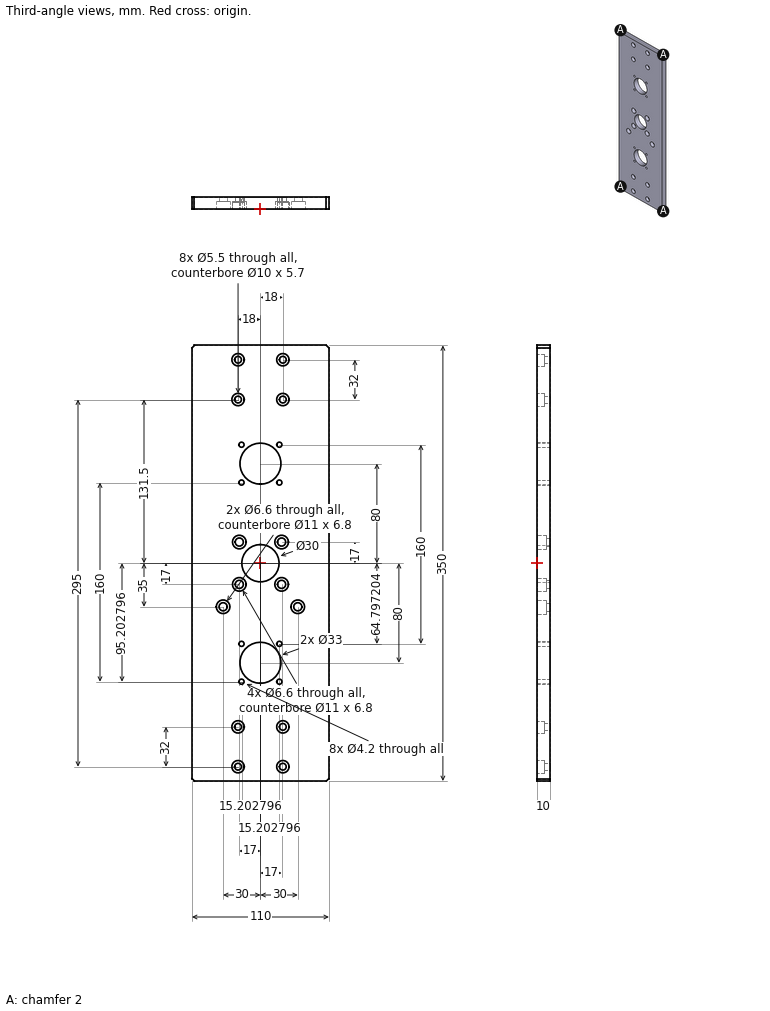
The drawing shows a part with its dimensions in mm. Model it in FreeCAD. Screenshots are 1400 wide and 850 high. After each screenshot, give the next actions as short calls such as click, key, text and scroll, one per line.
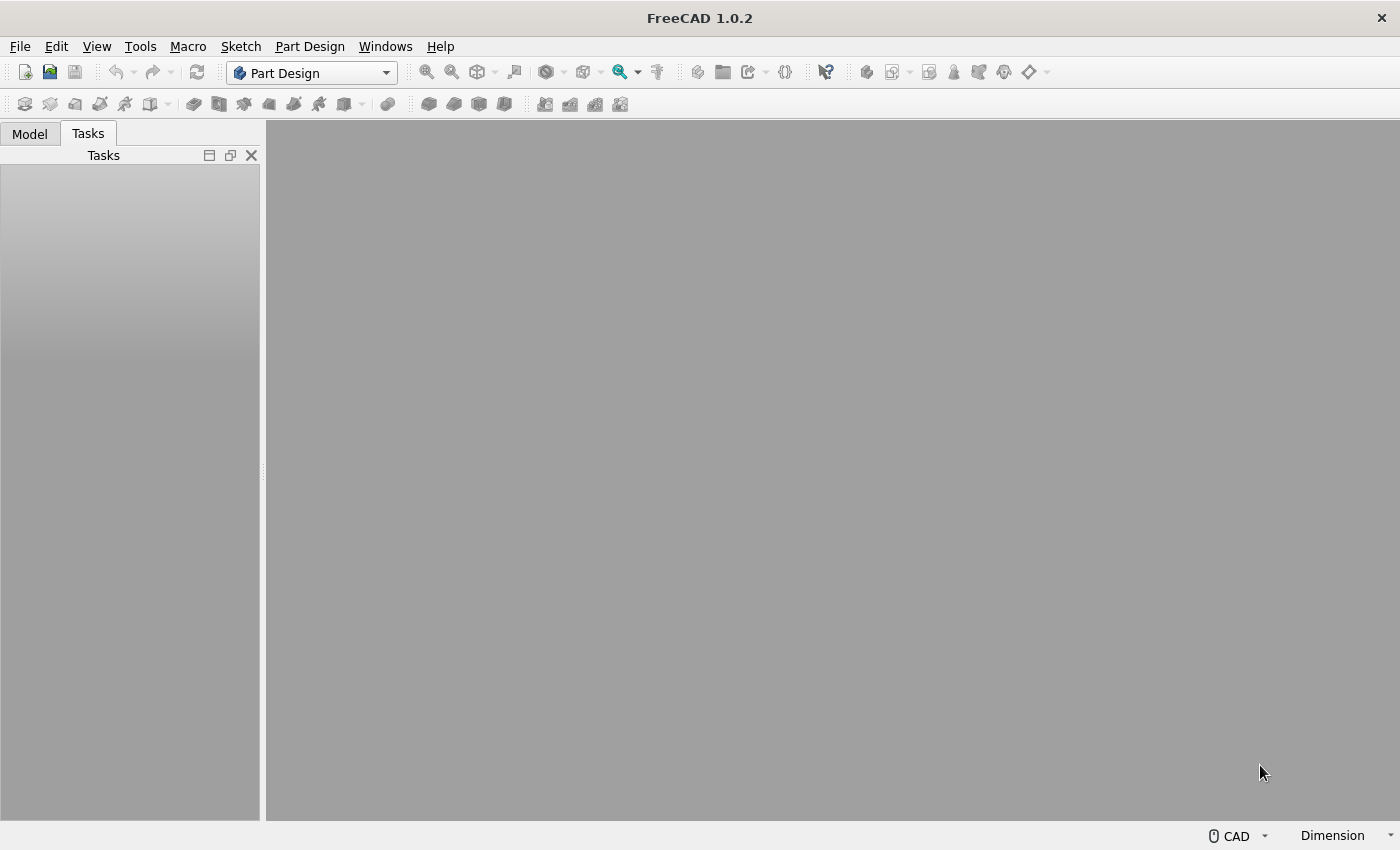
key(ctrl+n)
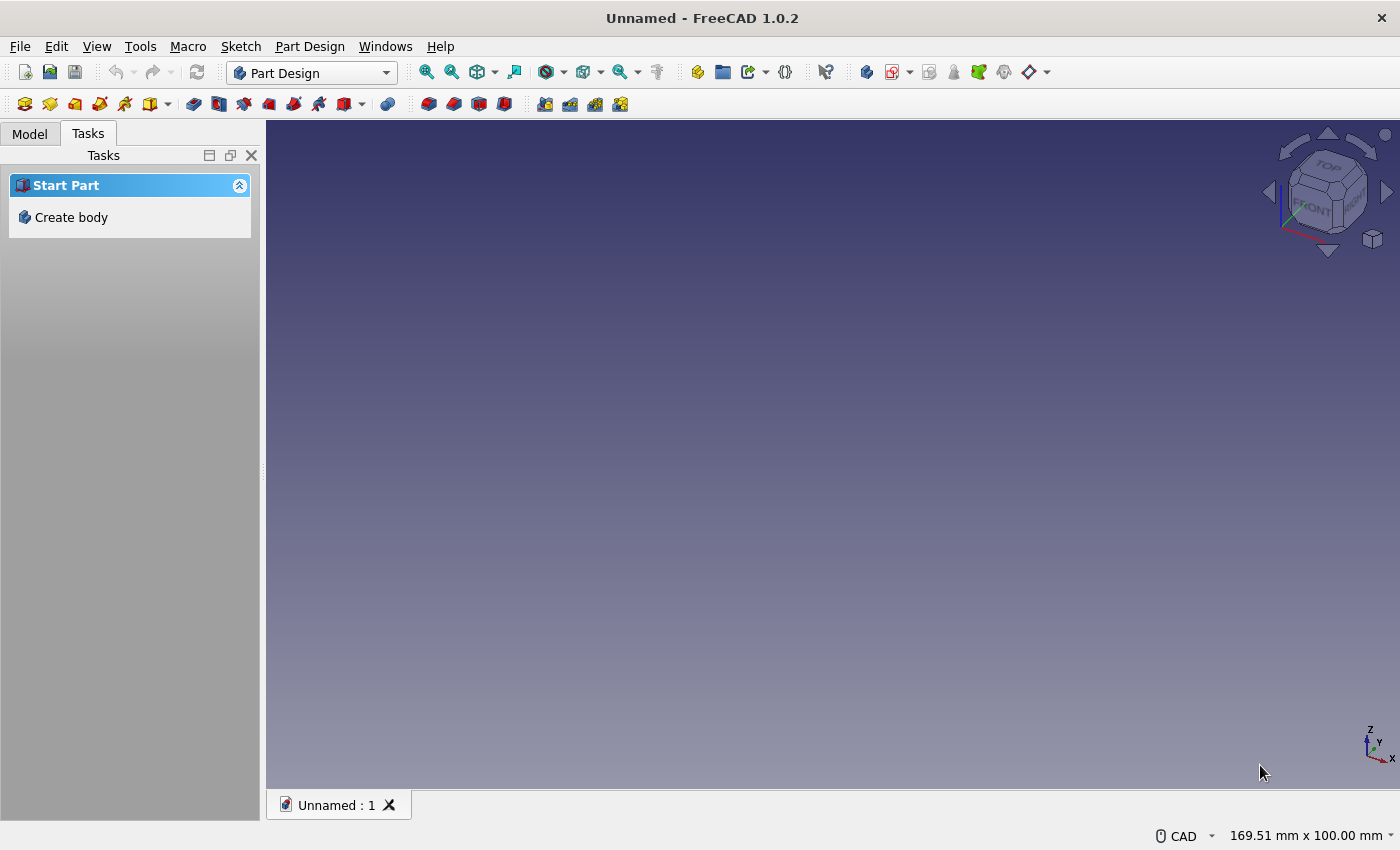
click(892, 72)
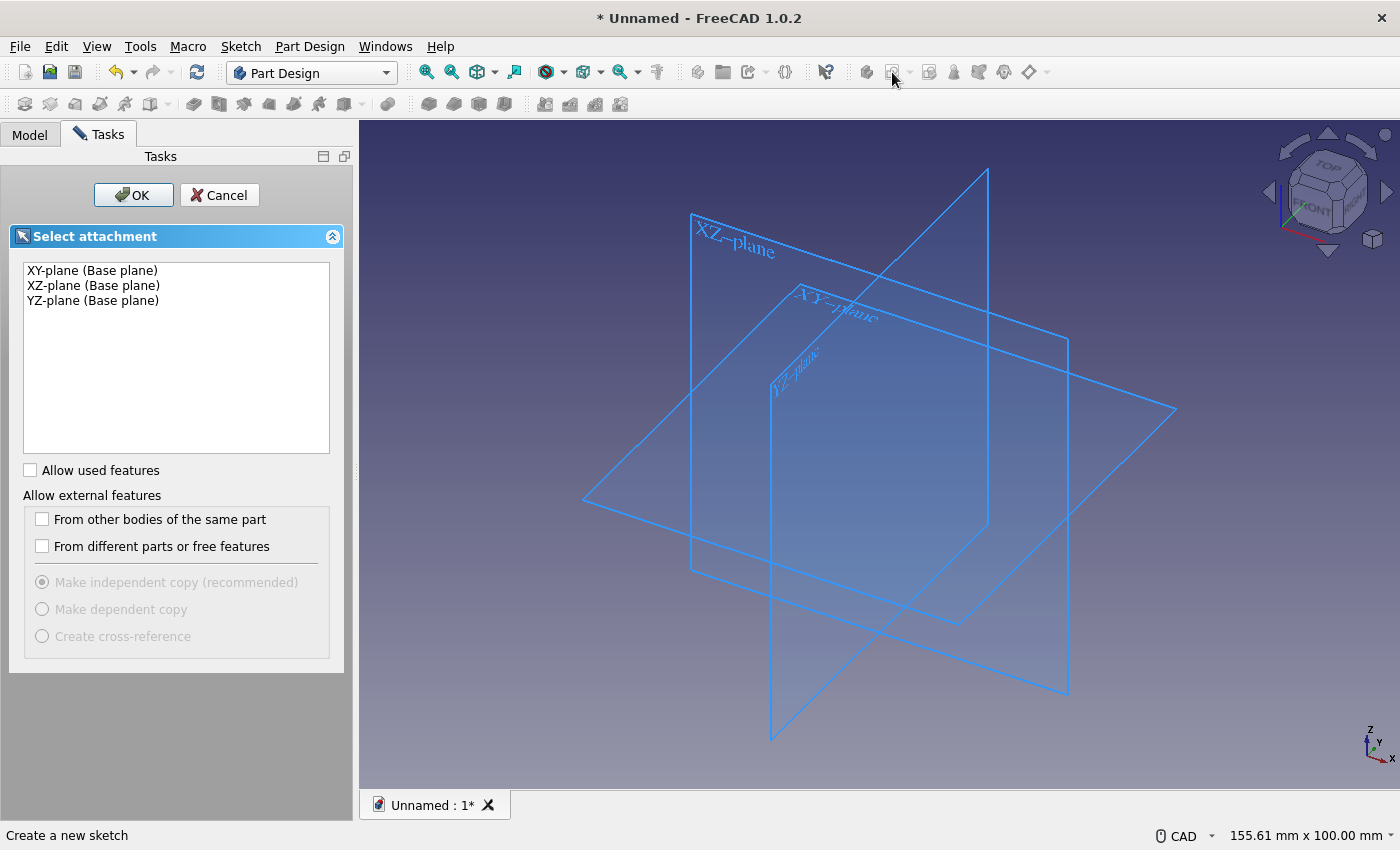
click(84, 286)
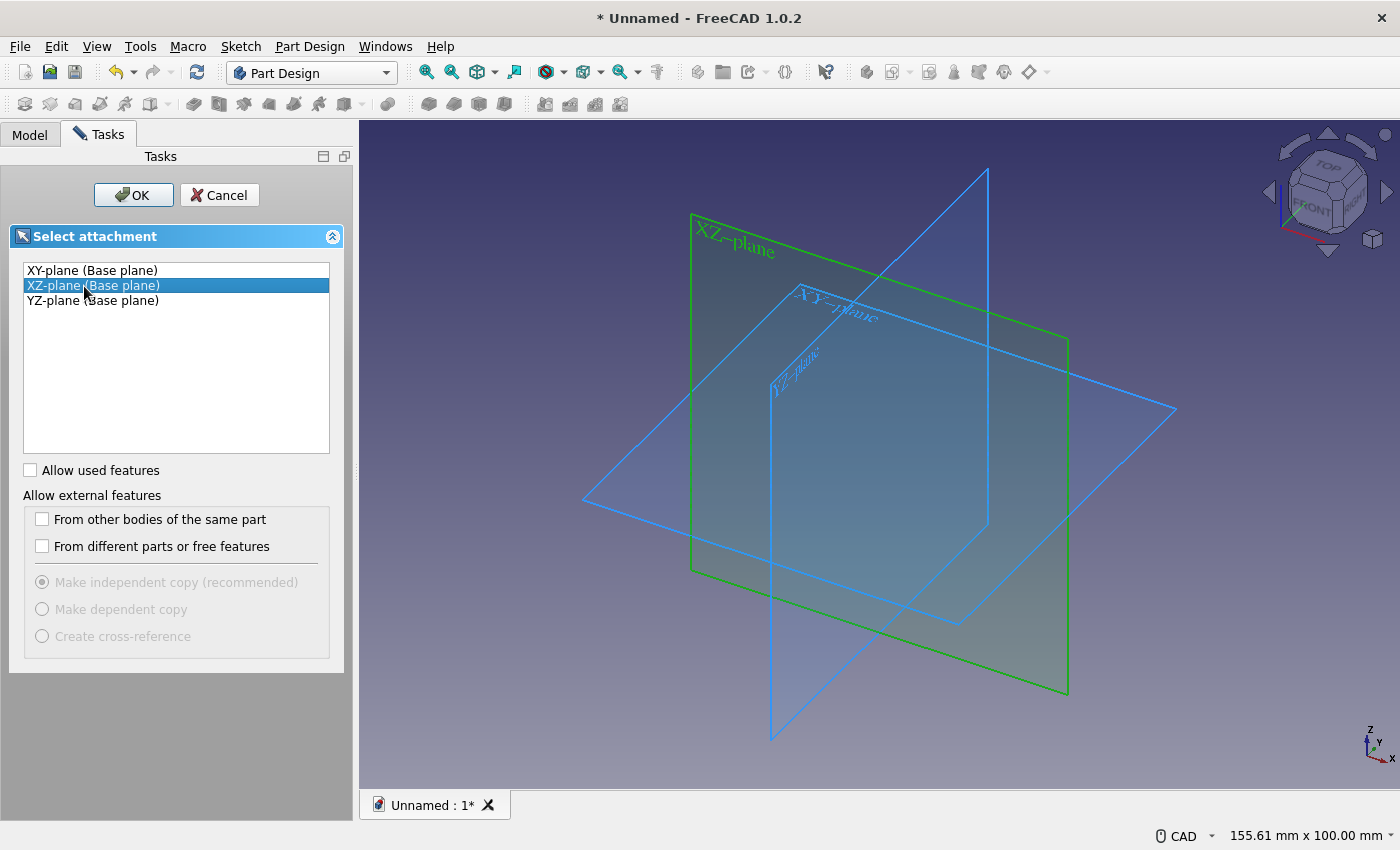
click(134, 195)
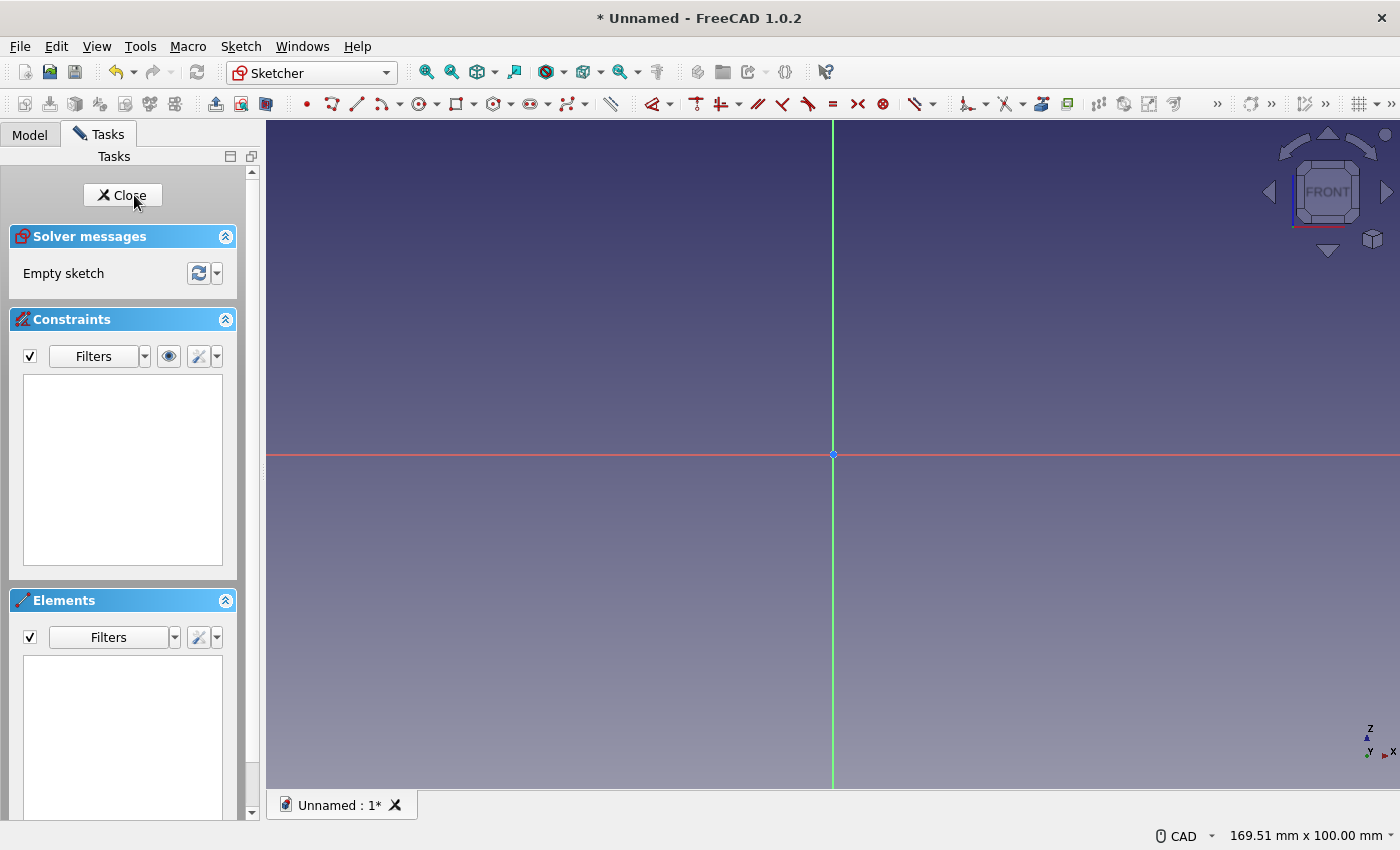
scroll(747, 454, down, 8)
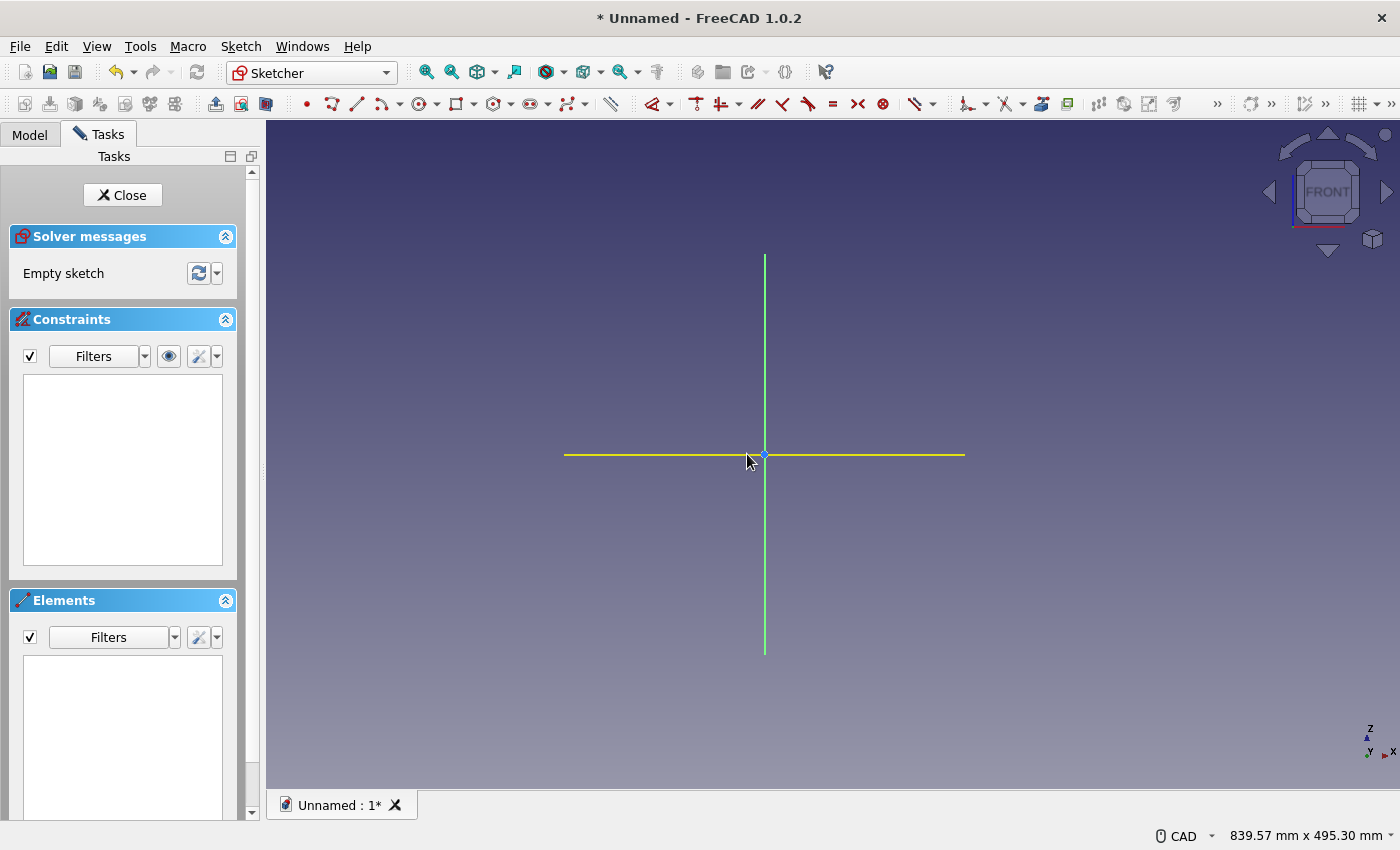
key(g)
key(v)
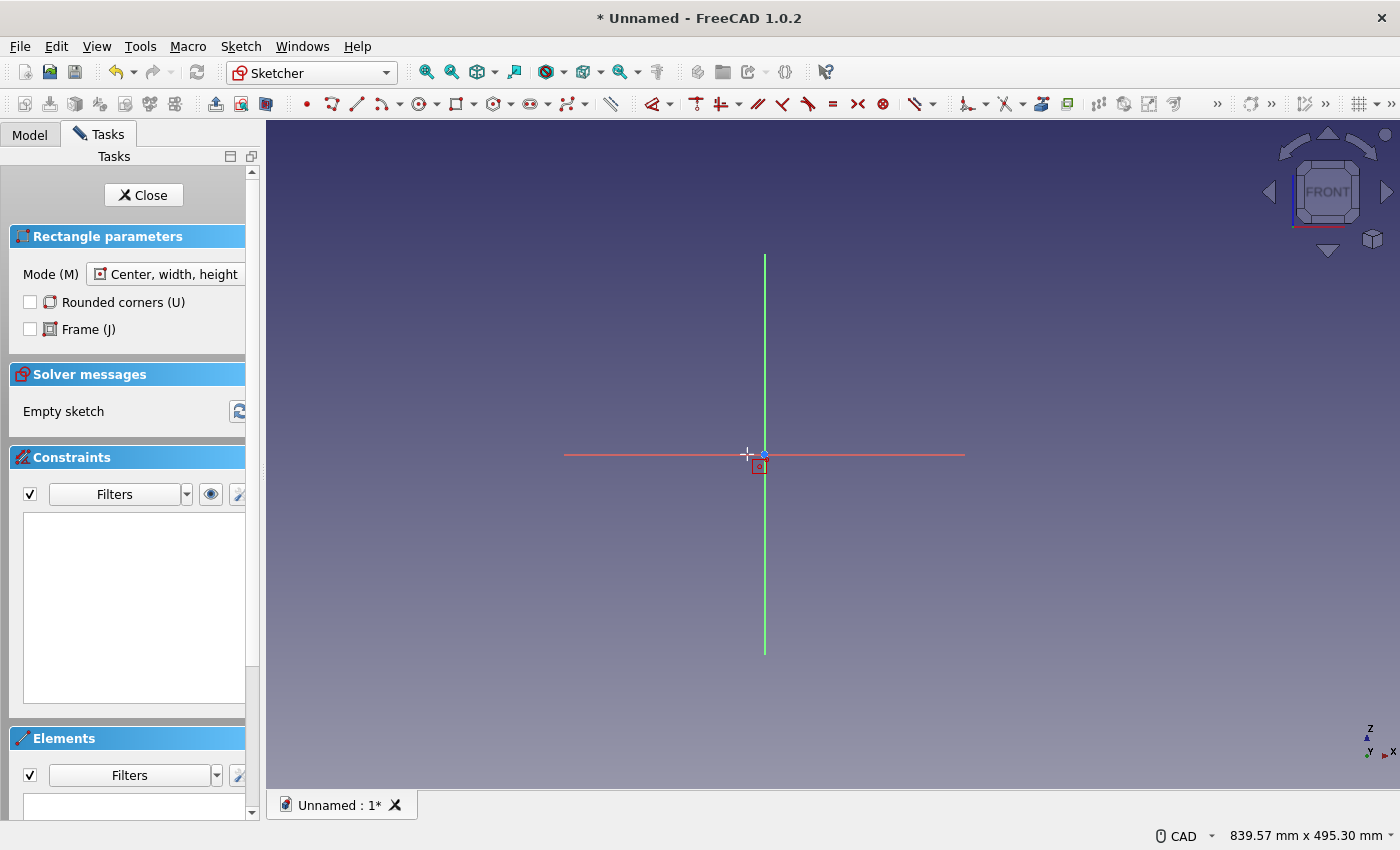
click(765, 454)
move(839, 218)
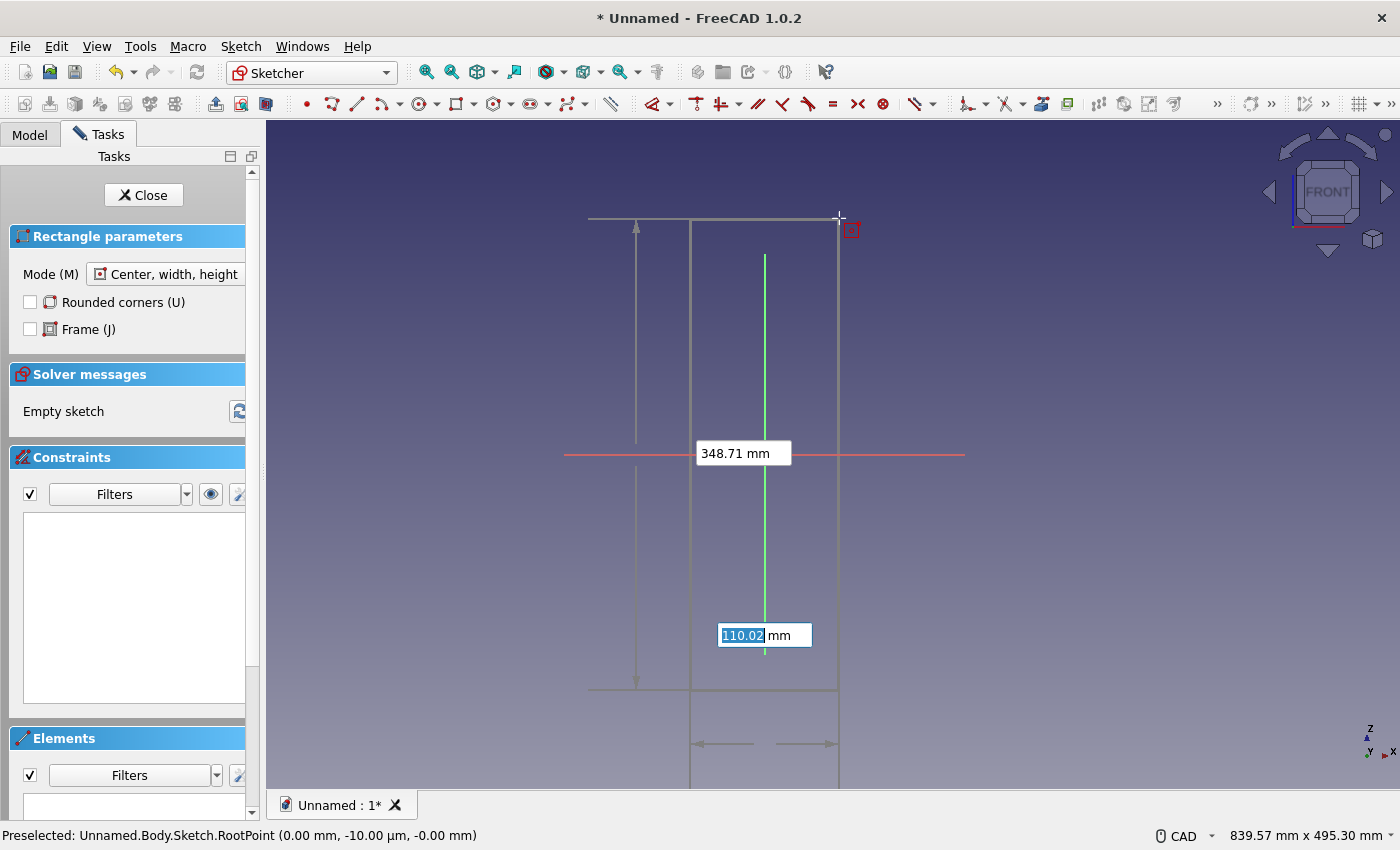
text(110)
key(Tab)
text(350)
key(Return)
key(Escape)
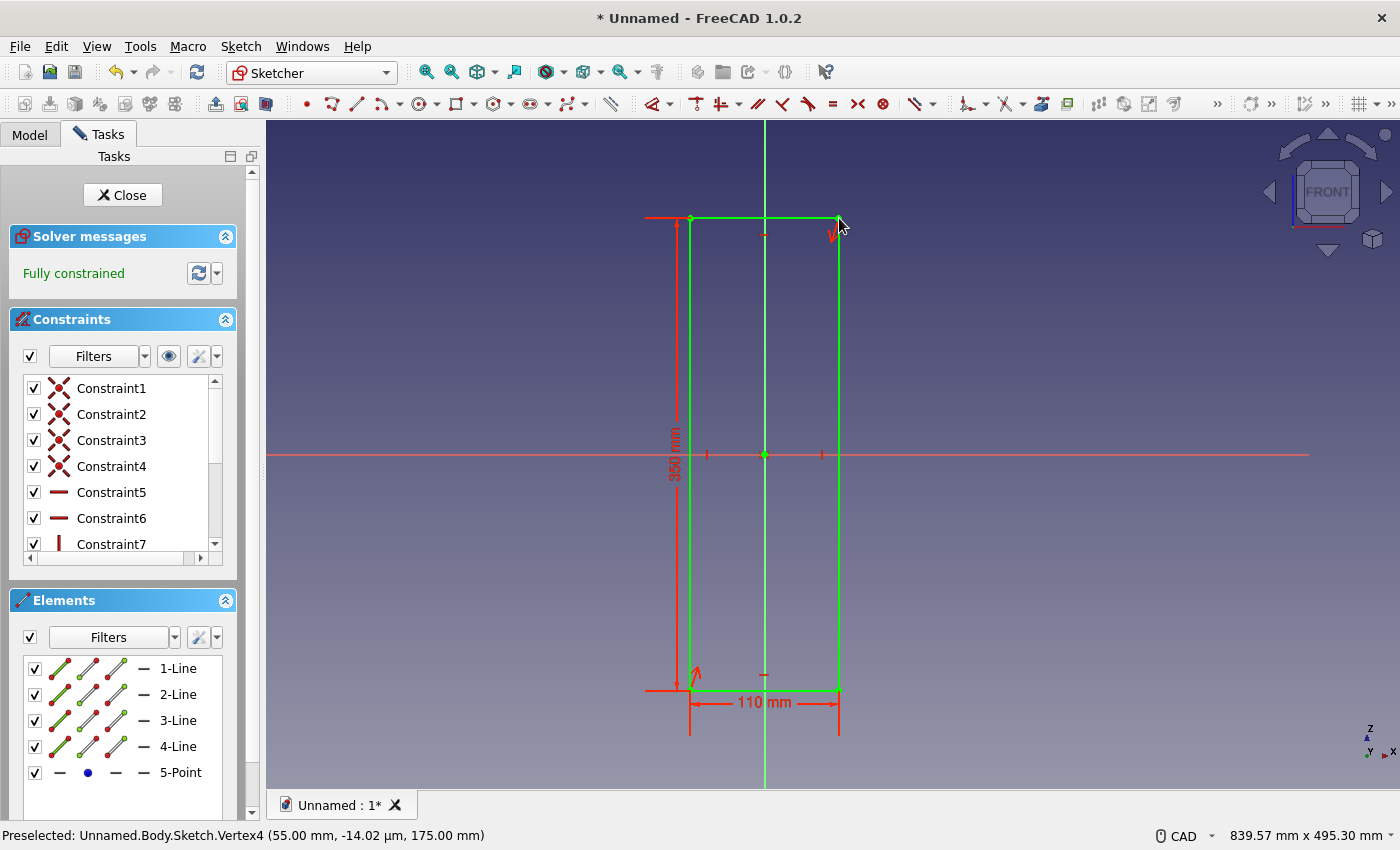
click(123, 195)